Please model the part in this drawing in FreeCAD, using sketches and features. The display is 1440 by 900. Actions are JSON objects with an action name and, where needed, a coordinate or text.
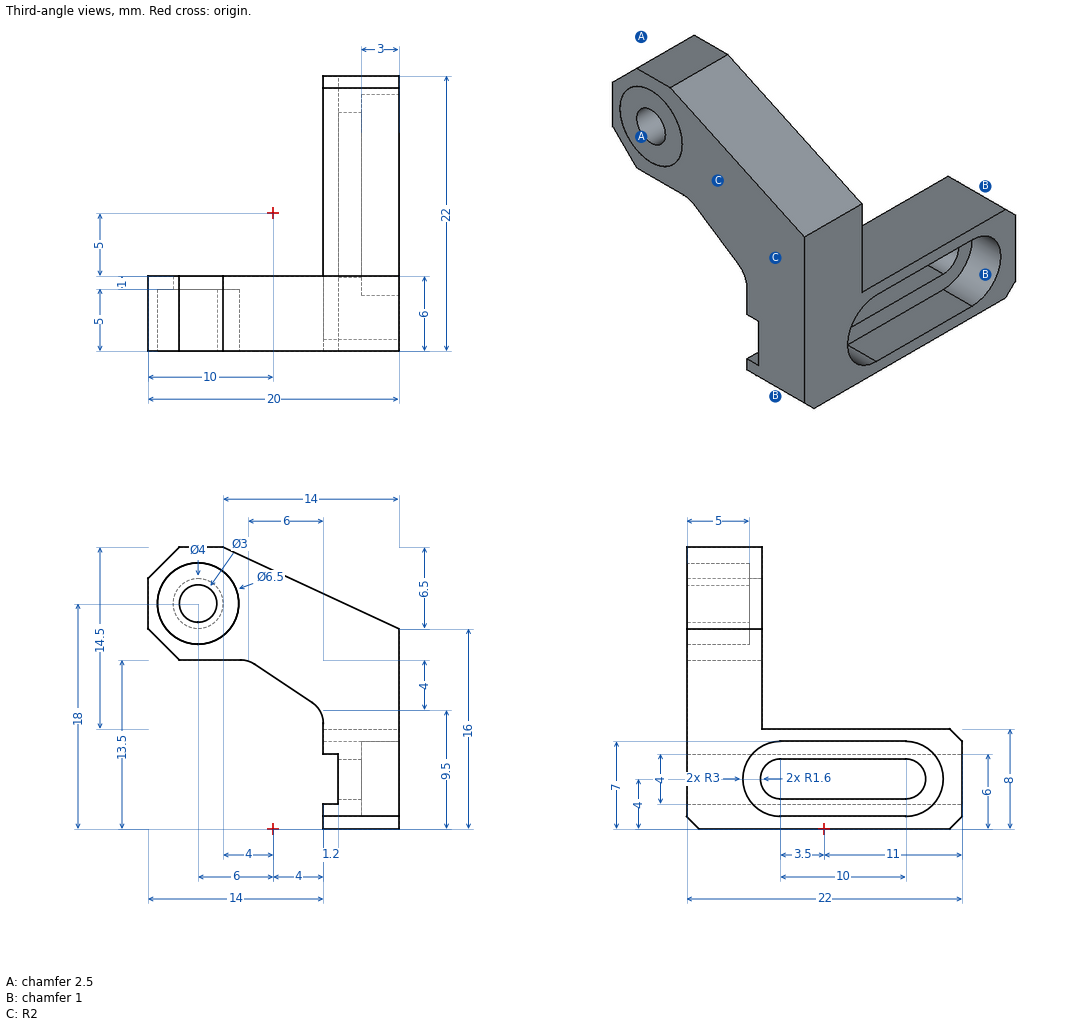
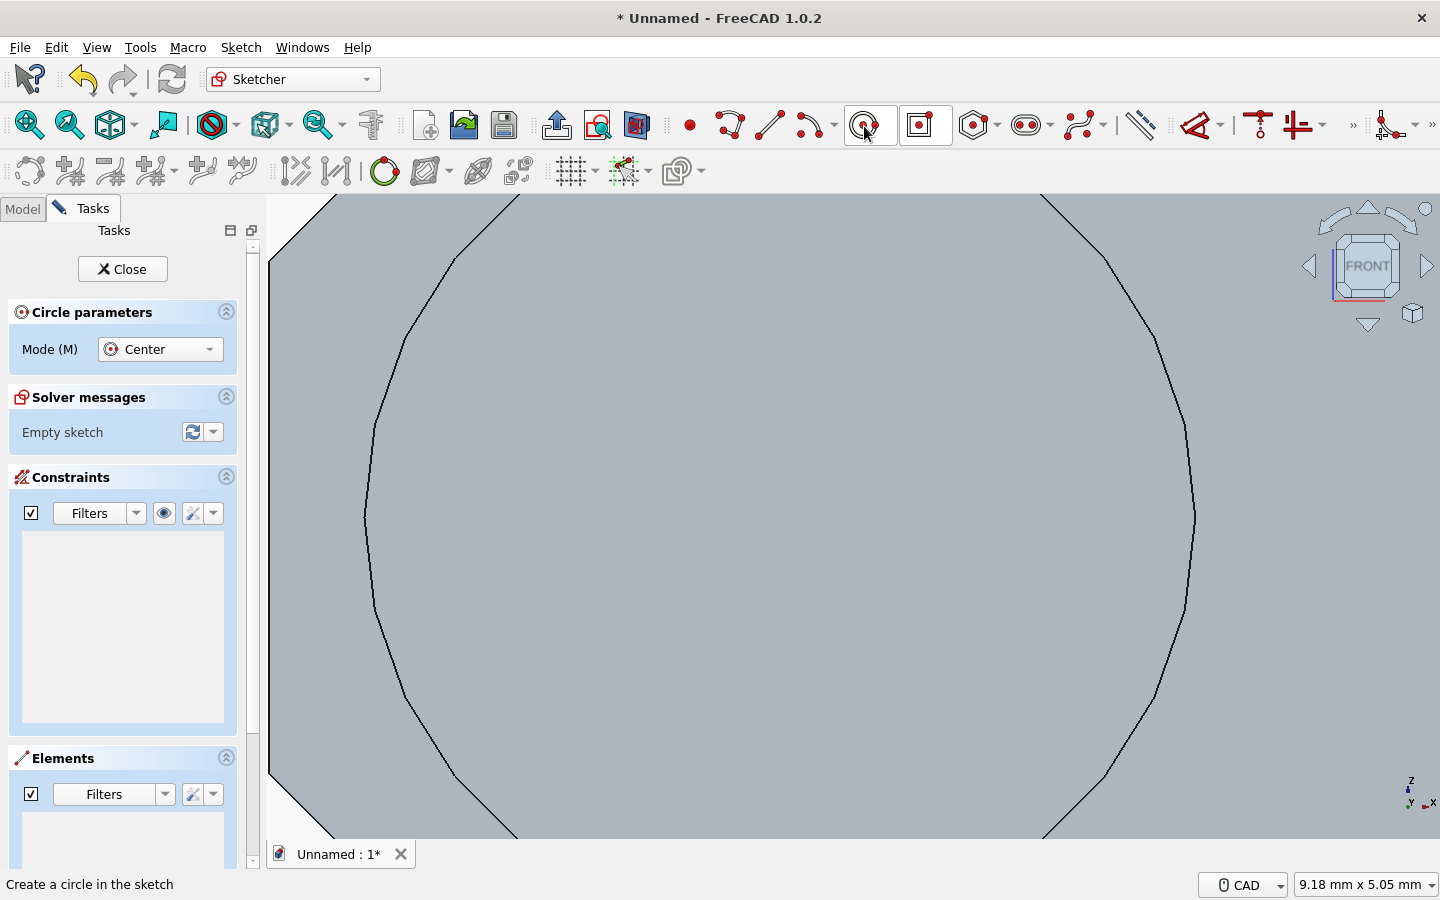
{"action": "left_click", "coordinate": [780, 518]}
{"action": "mouse_move", "coordinate": [915, 382]}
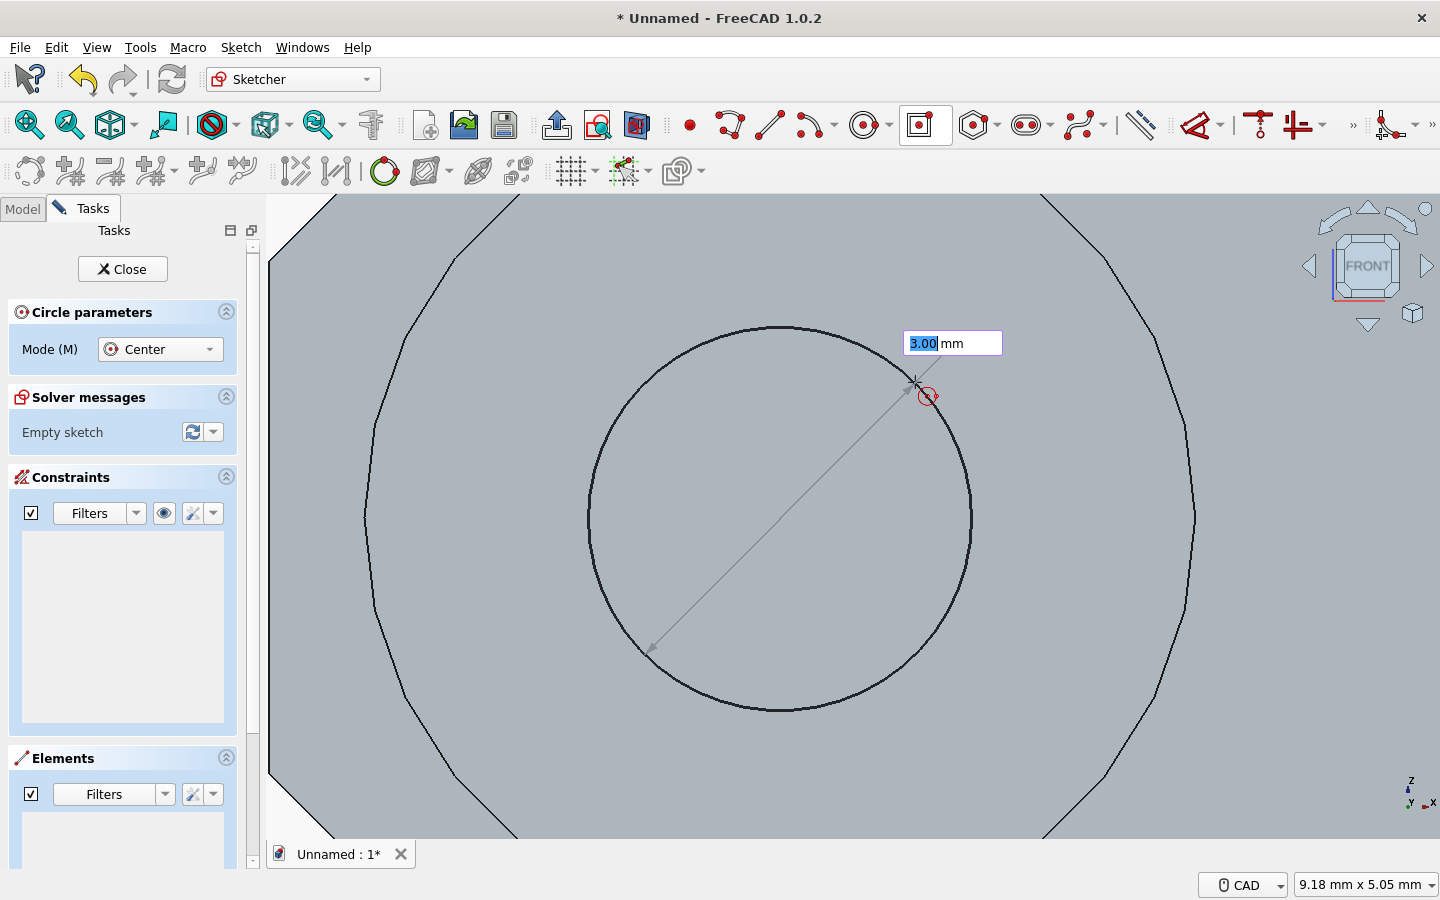
{"action": "type", "text": "3"}
{"action": "key", "text": "Return"}
{"action": "key", "text": "Escape"}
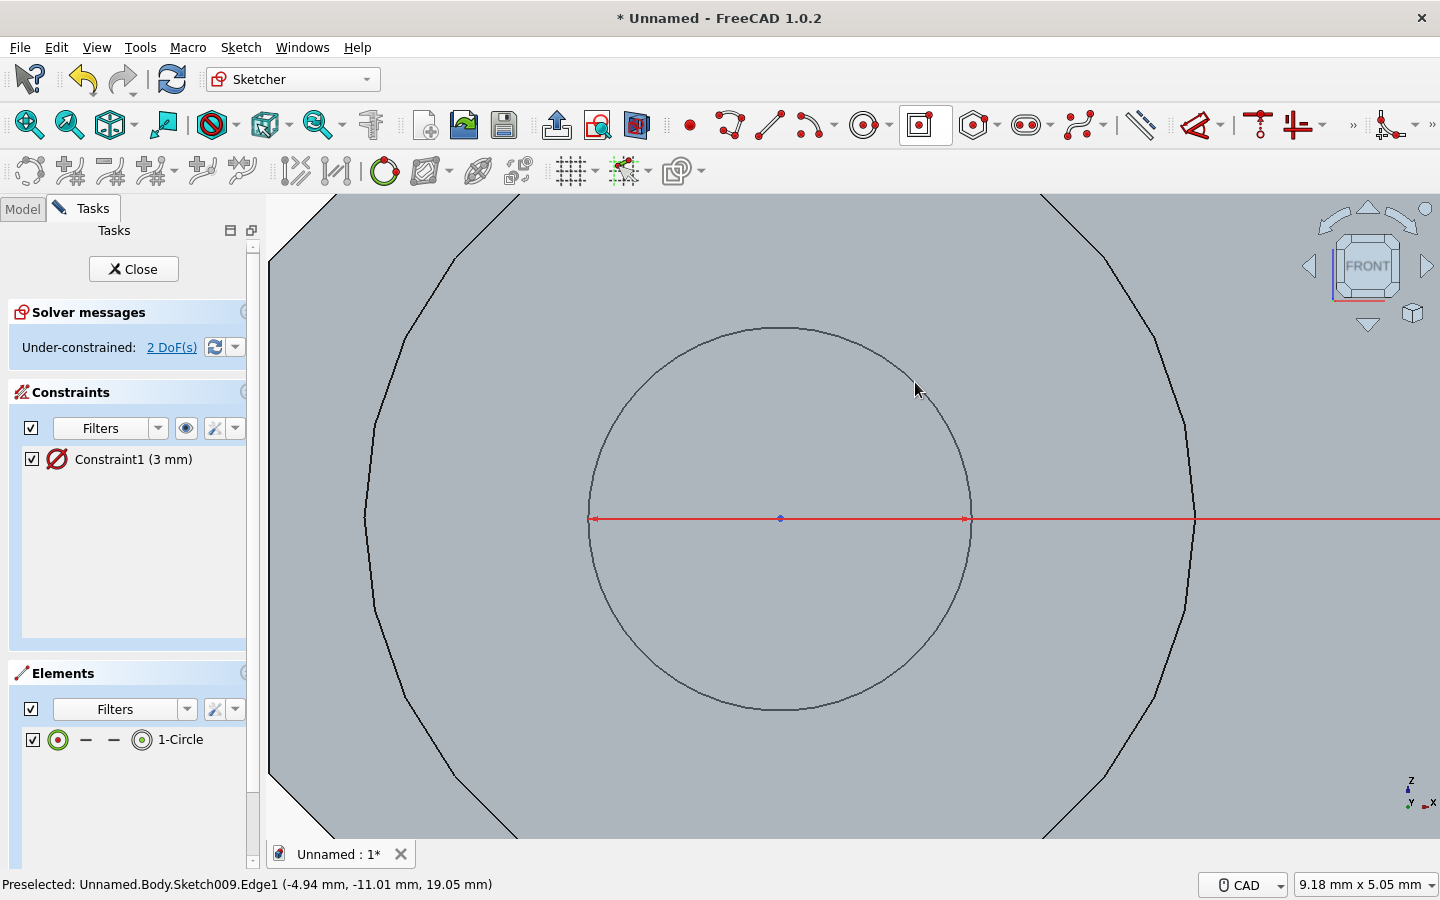
{"action": "left_click", "coordinate": [1196, 126]}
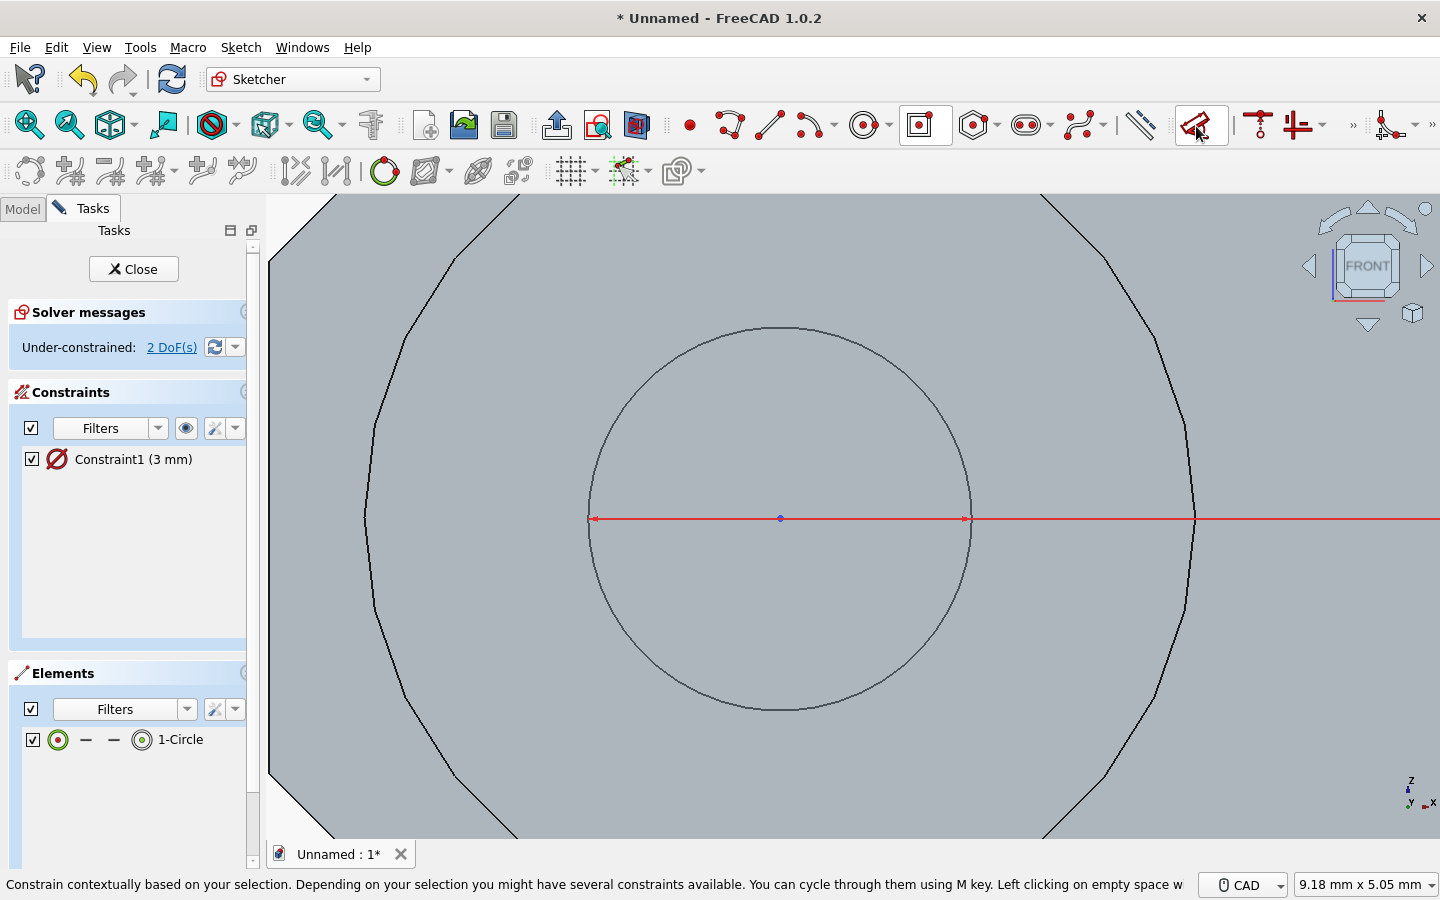
{"action": "left_click", "coordinate": [780, 519]}
{"action": "left_click", "coordinate": [1027, 485]}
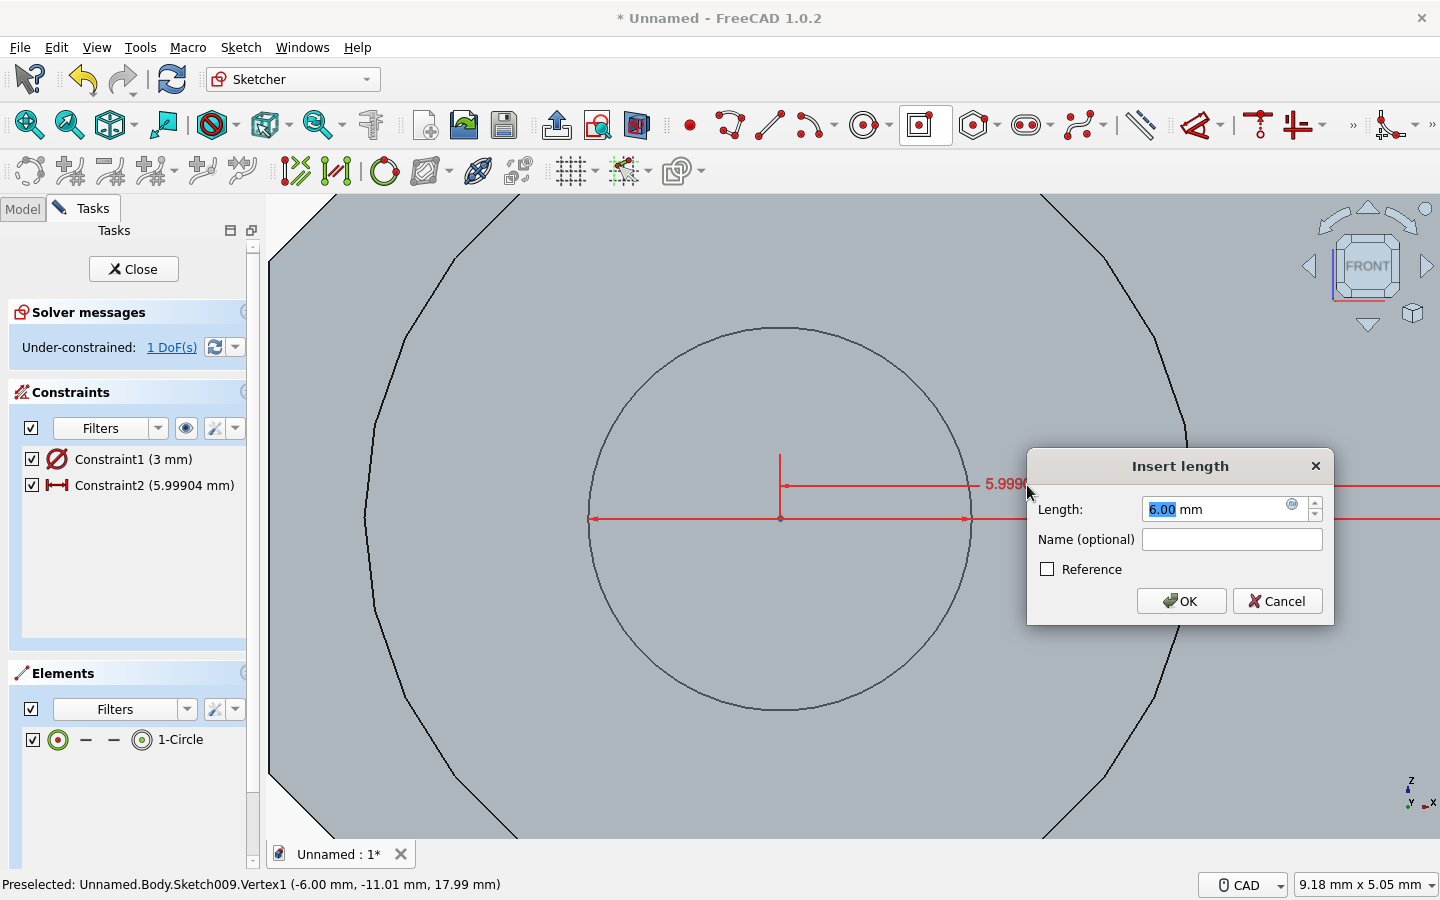
{"action": "type", "text": "6"}
{"action": "key", "text": "Return"}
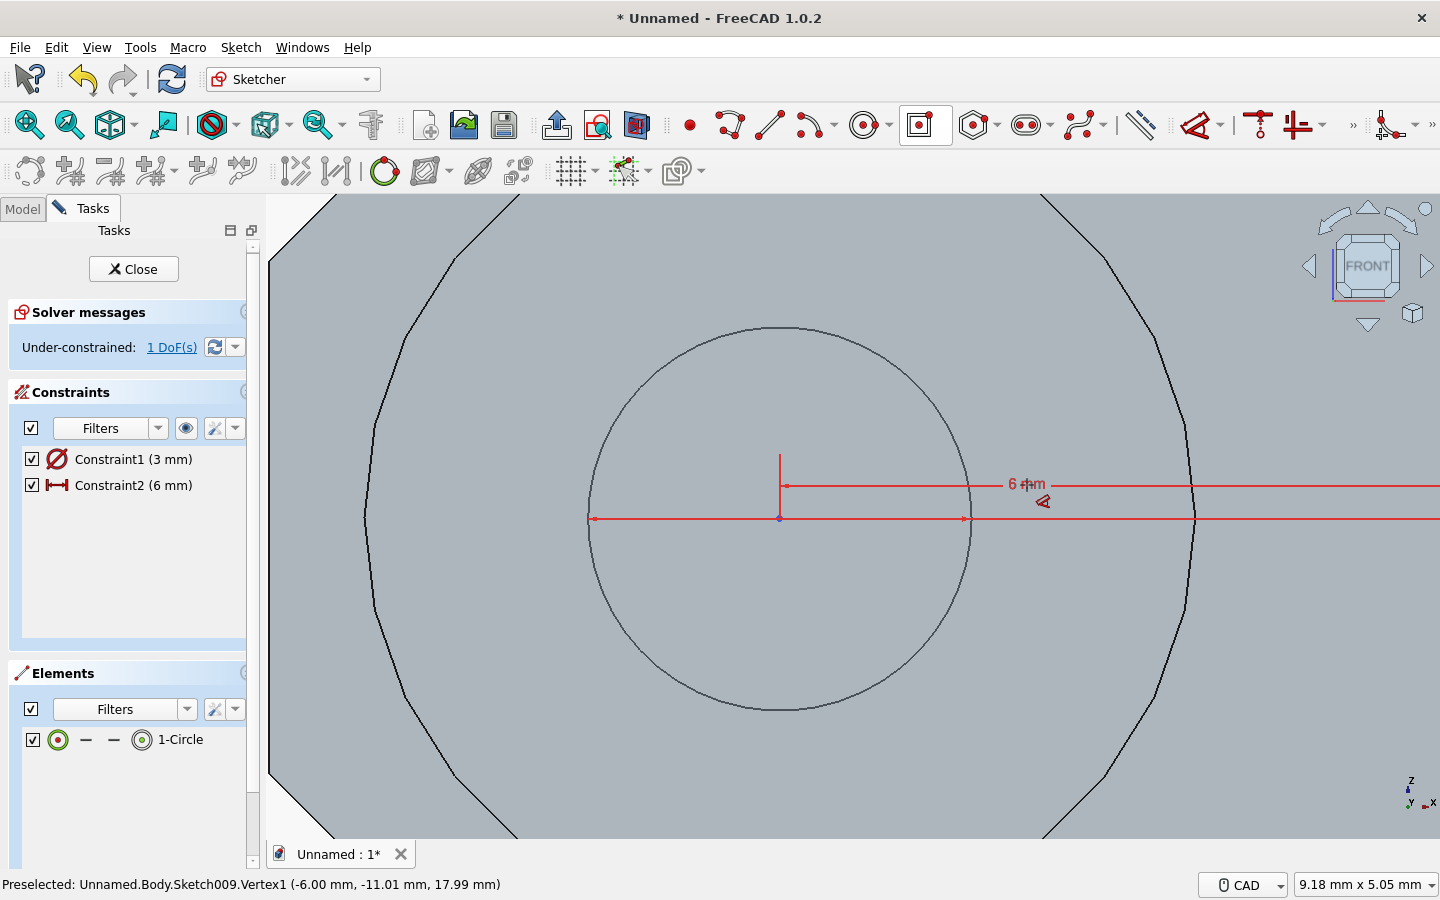
{"action": "left_click", "coordinate": [780, 519]}
{"action": "left_click", "coordinate": [746, 665]}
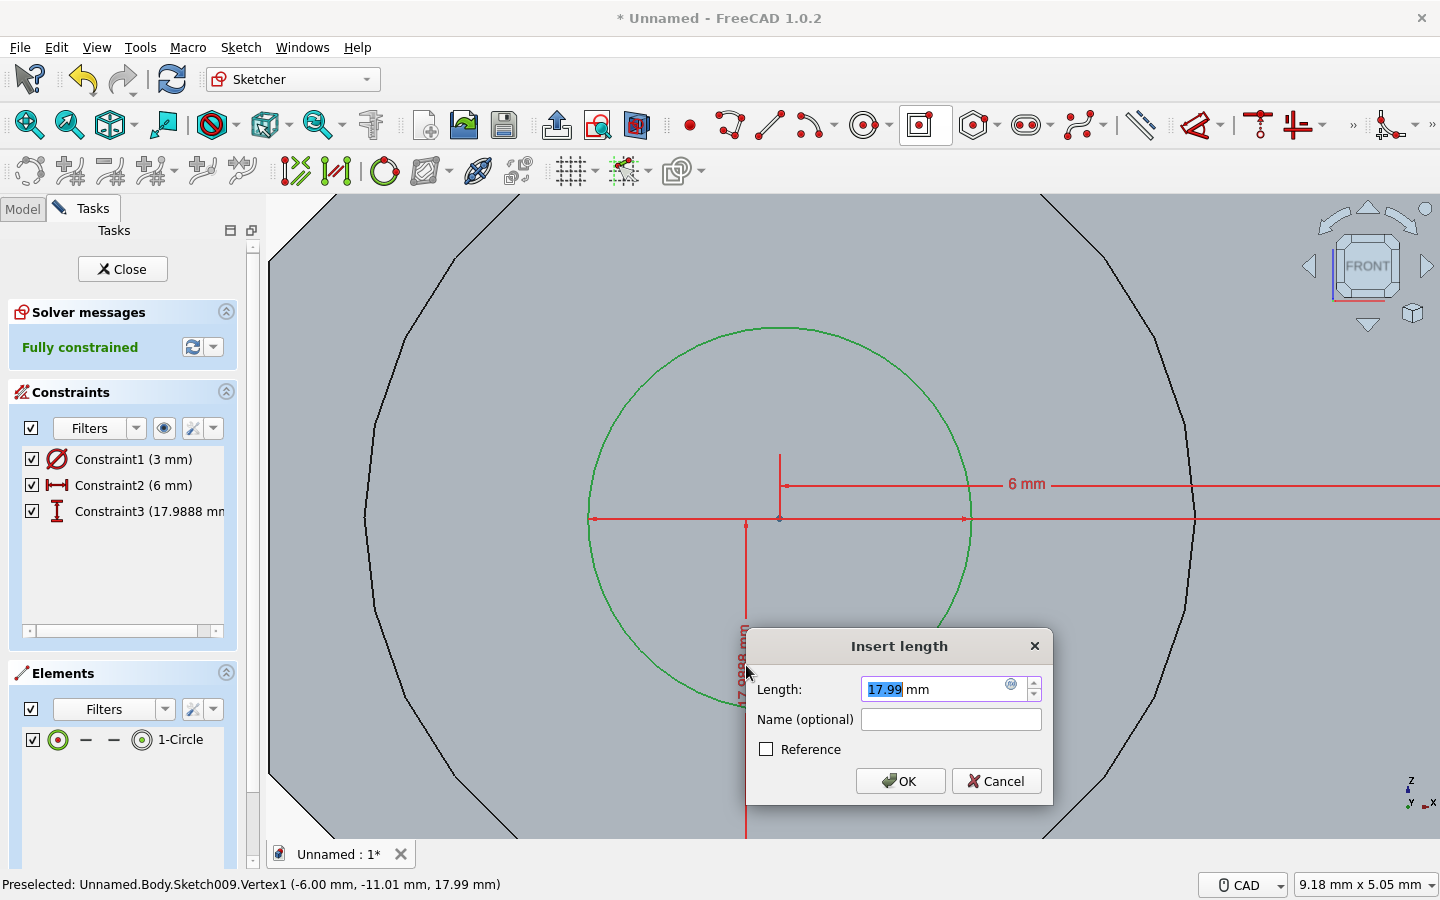
{"action": "type", "text": "18"}
{"action": "key", "text": "Return"}
{"action": "key", "text": "Escape"}